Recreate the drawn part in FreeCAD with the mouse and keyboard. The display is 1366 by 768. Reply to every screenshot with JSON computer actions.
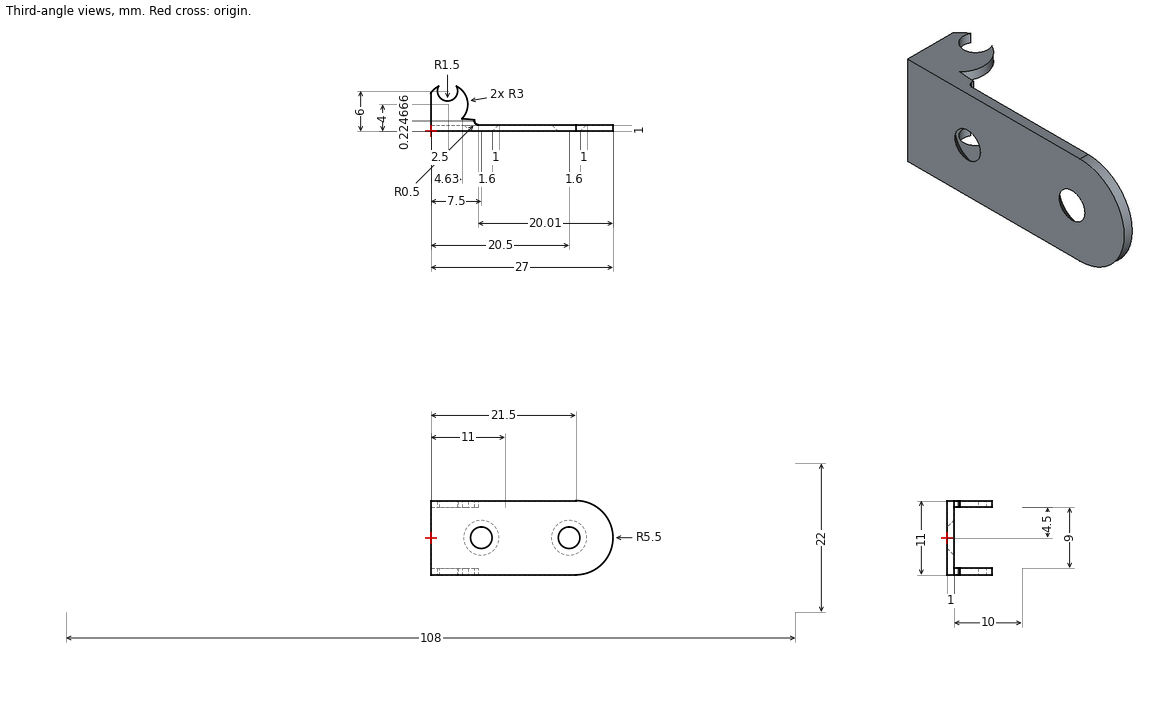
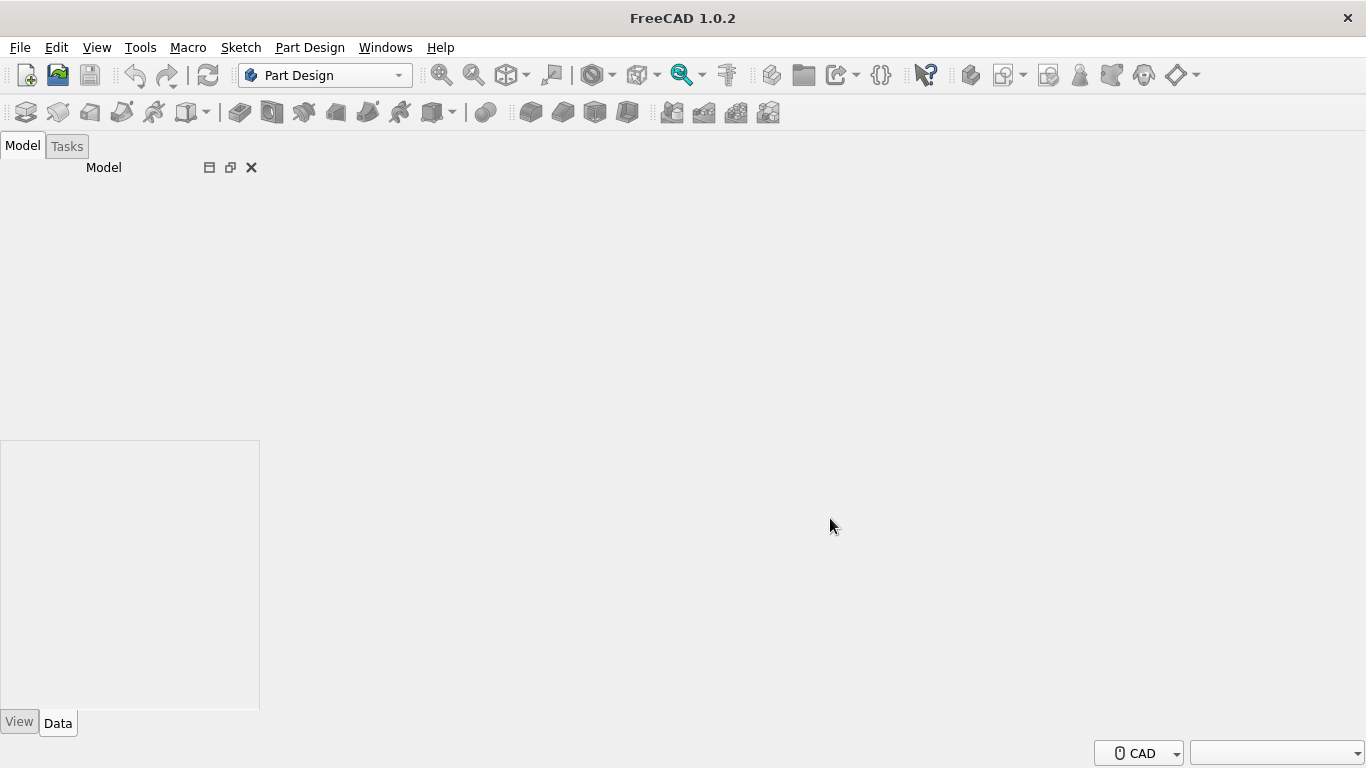
{"action": "left_click", "coordinate": [26, 76]}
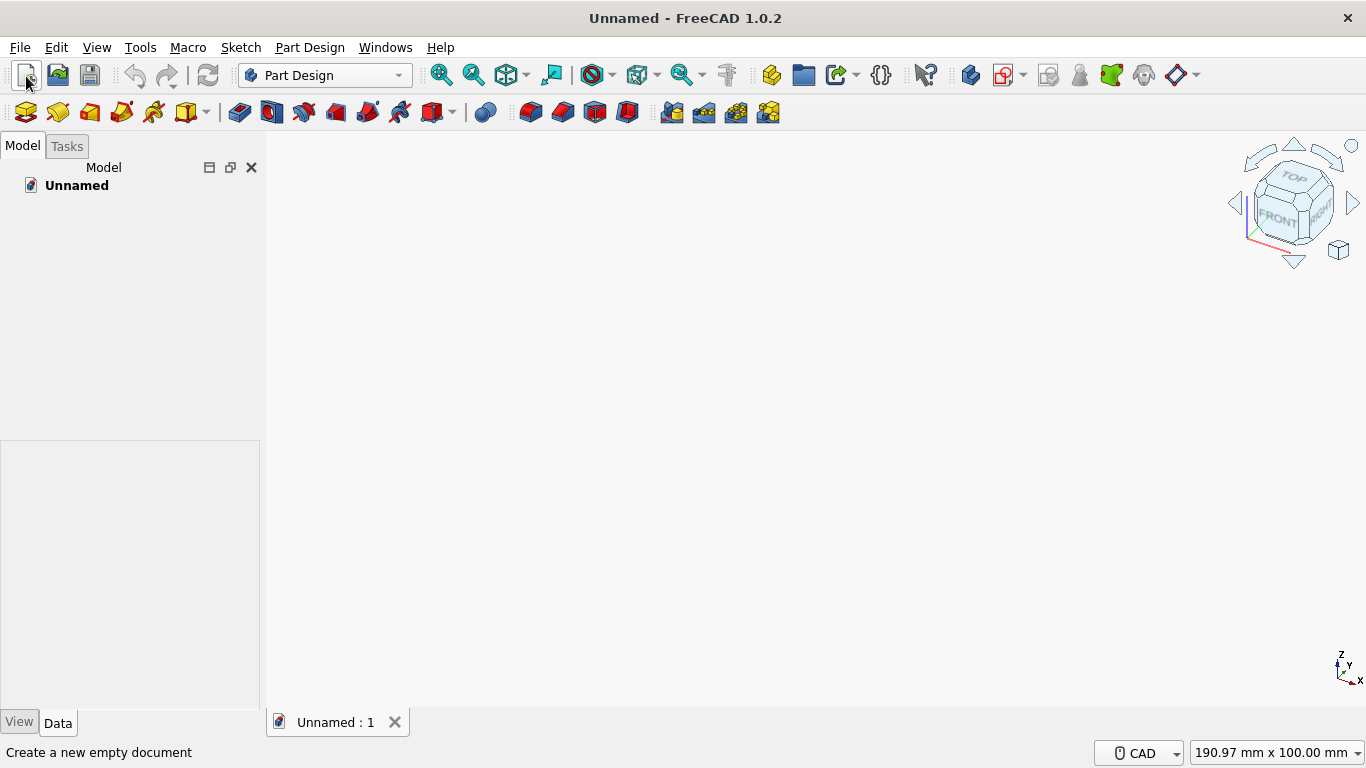
{"action": "left_click", "coordinate": [1004, 76]}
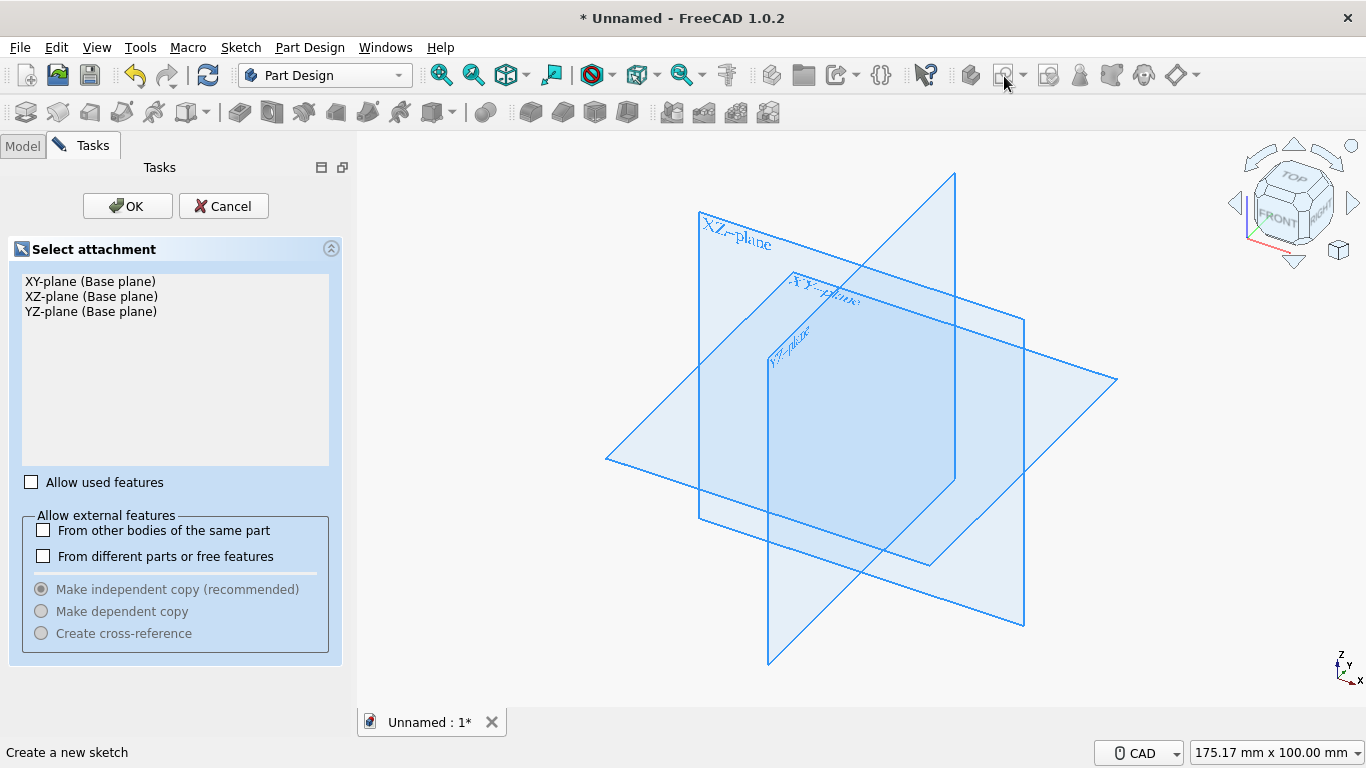
{"action": "left_click", "coordinate": [82, 282]}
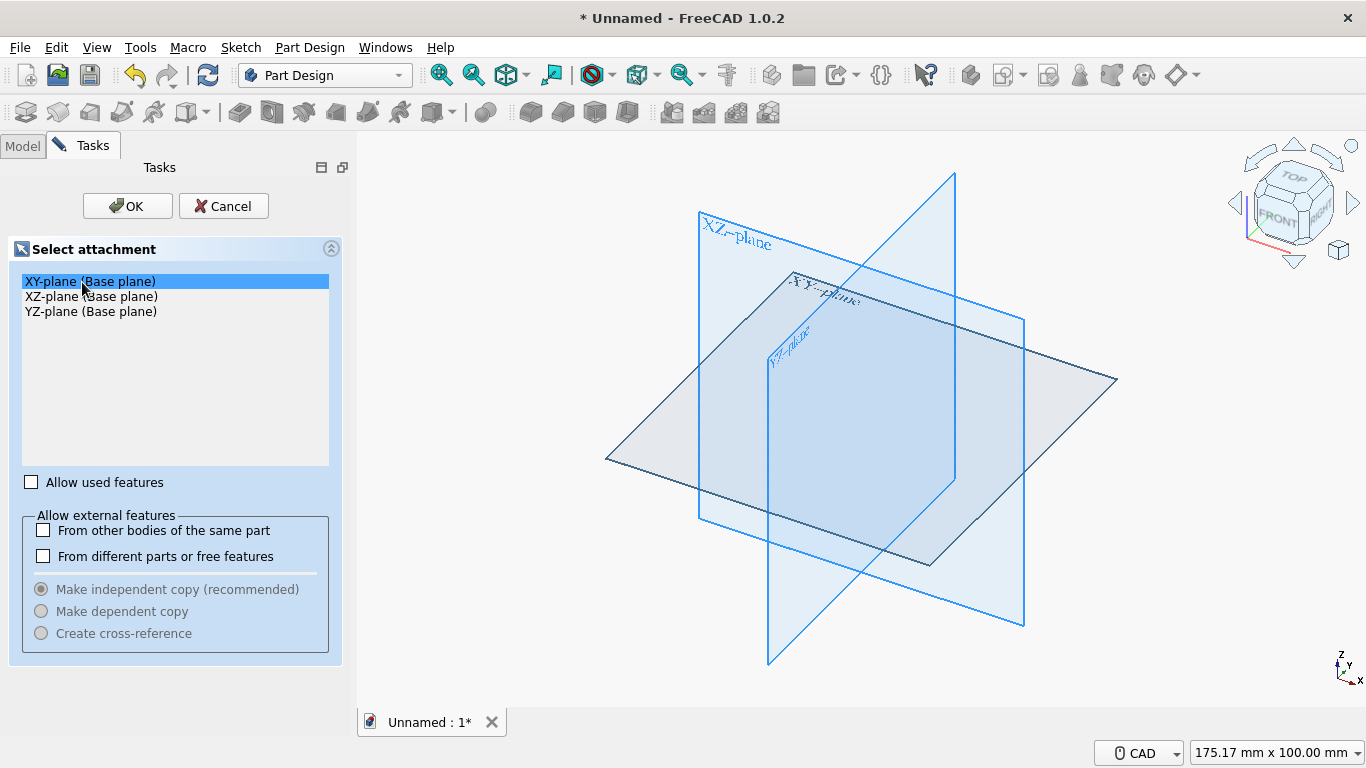
{"action": "left_click", "coordinate": [128, 206]}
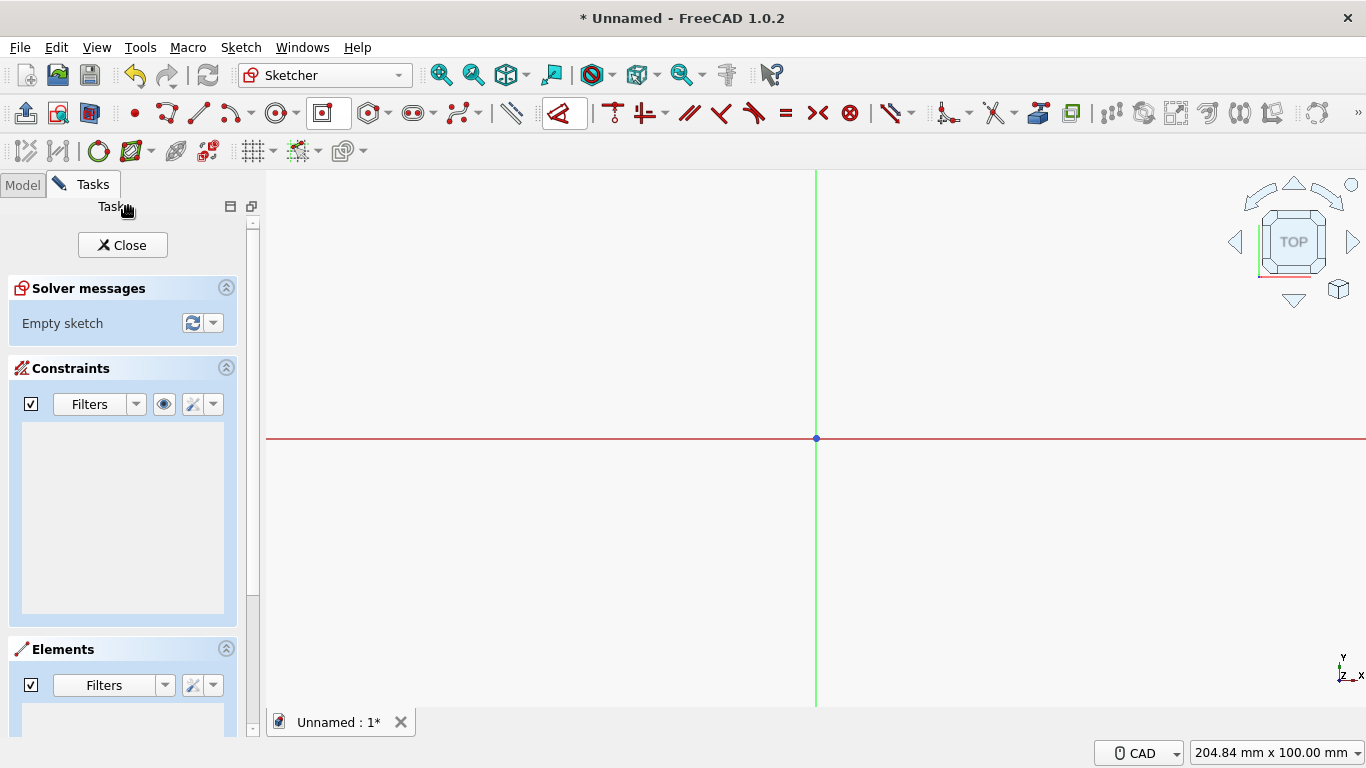
{"action": "scroll", "coordinate": [935, 415], "scroll_direction": "up", "scroll_amount": 7}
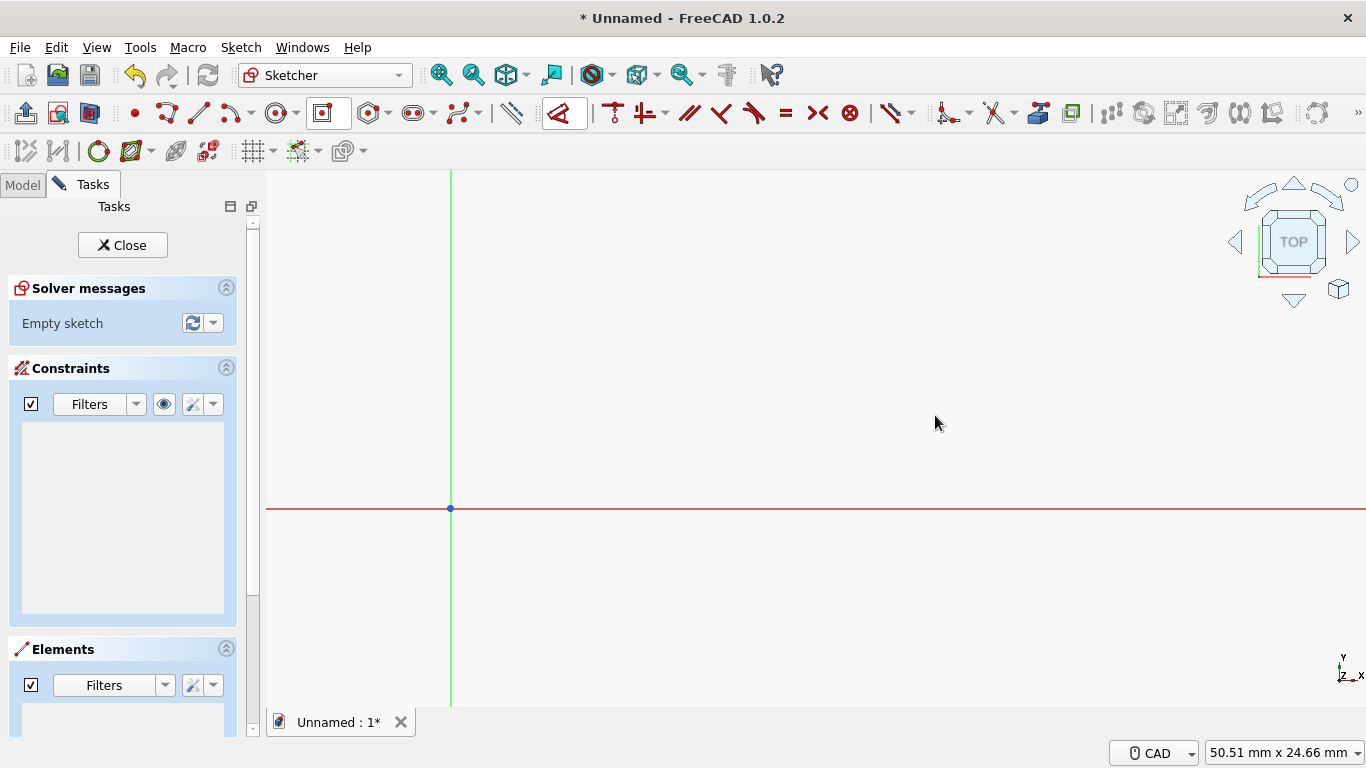
{"action": "left_click", "coordinate": [168, 114]}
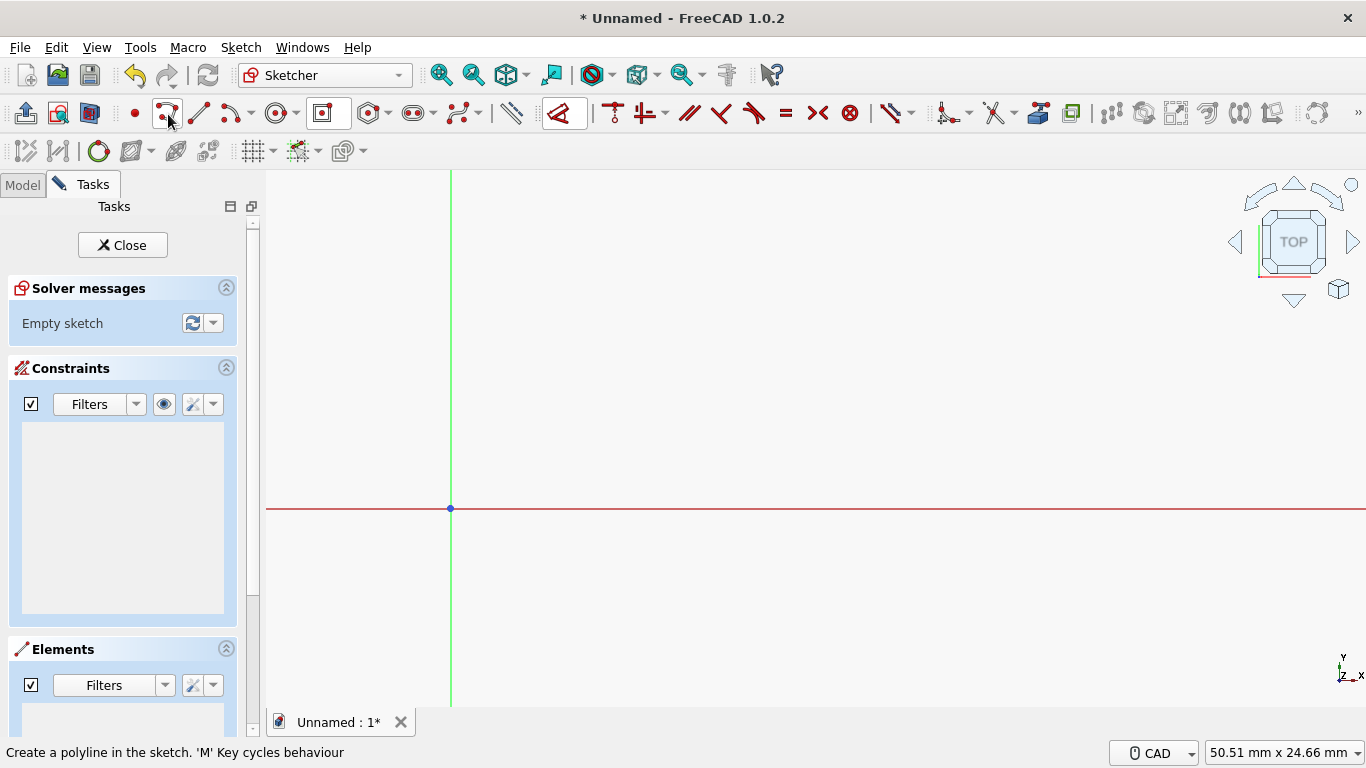
{"action": "left_click", "coordinate": [592, 476]}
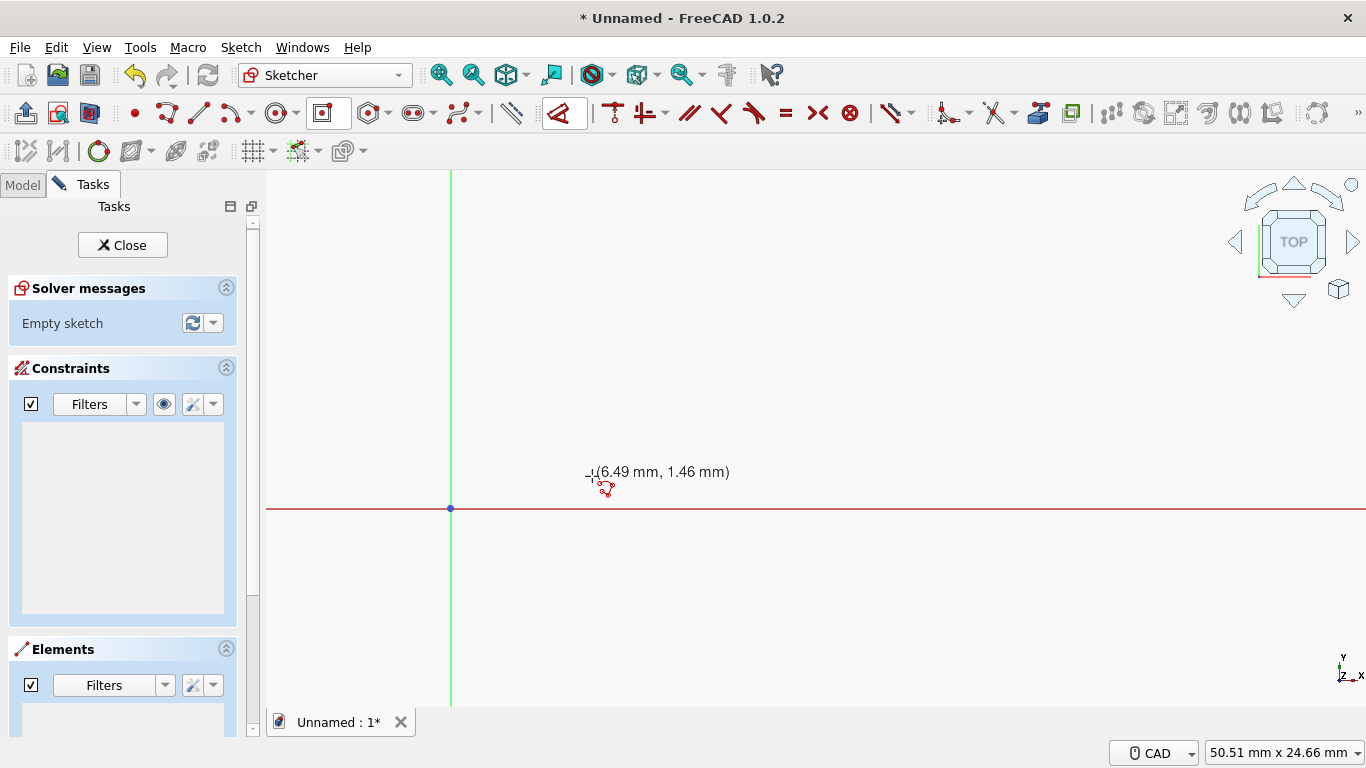
{"action": "scroll", "coordinate": [592, 471], "scroll_direction": "up", "scroll_amount": 6}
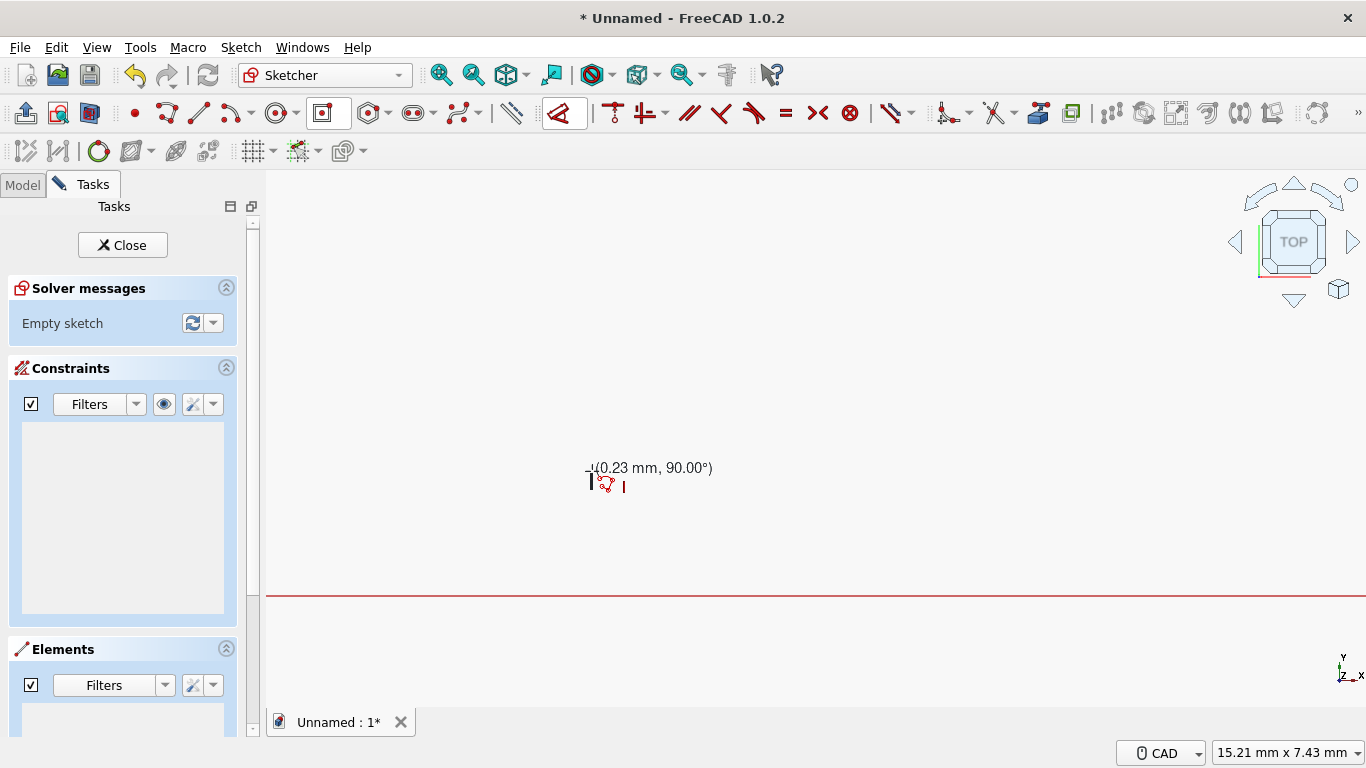
{"action": "left_click", "coordinate": [591, 471]}
{"action": "left_click", "coordinate": [457, 459]}
{"action": "right_click", "coordinate": [457, 459]}